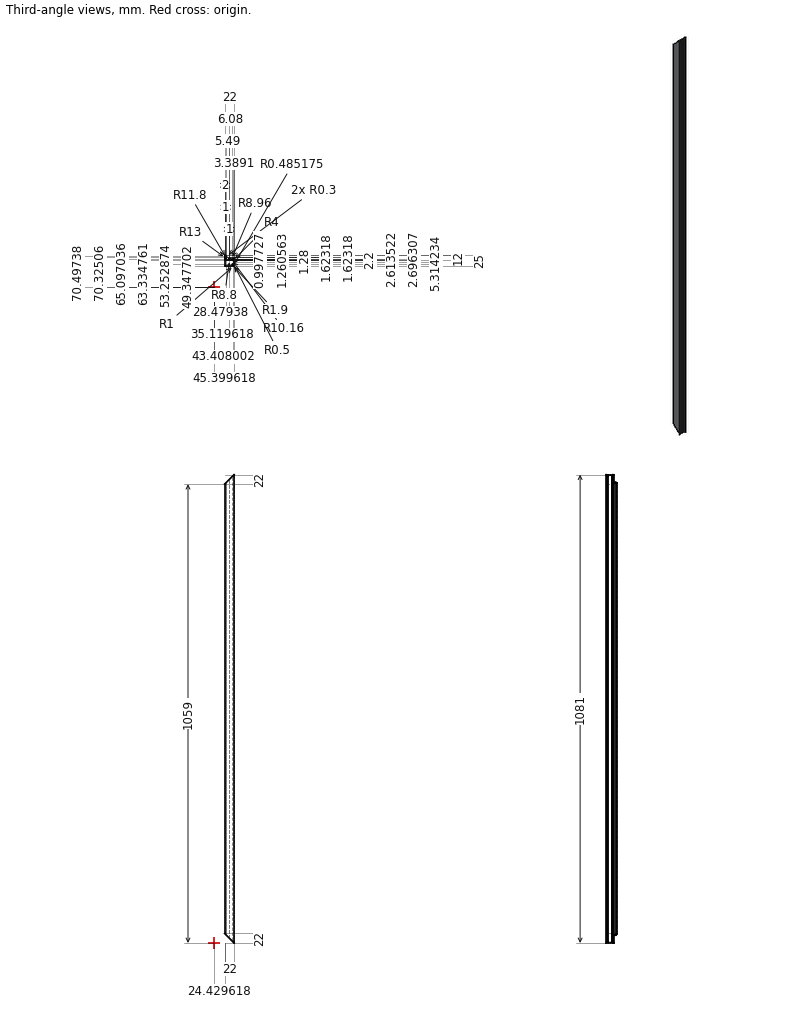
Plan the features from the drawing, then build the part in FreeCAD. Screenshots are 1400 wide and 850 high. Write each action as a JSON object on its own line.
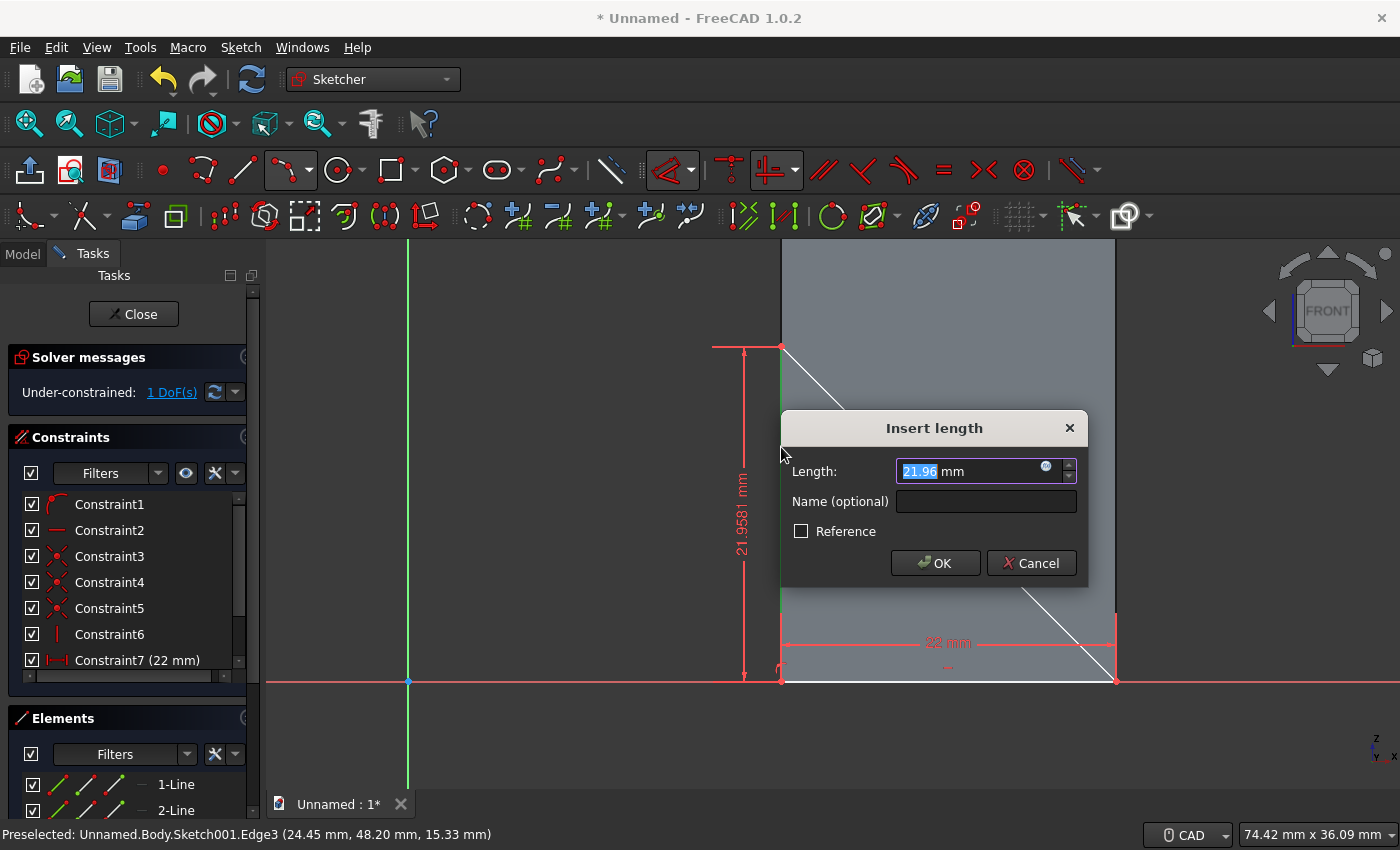
{"action": "type", "text": "22"}
{"action": "key", "text": "Return"}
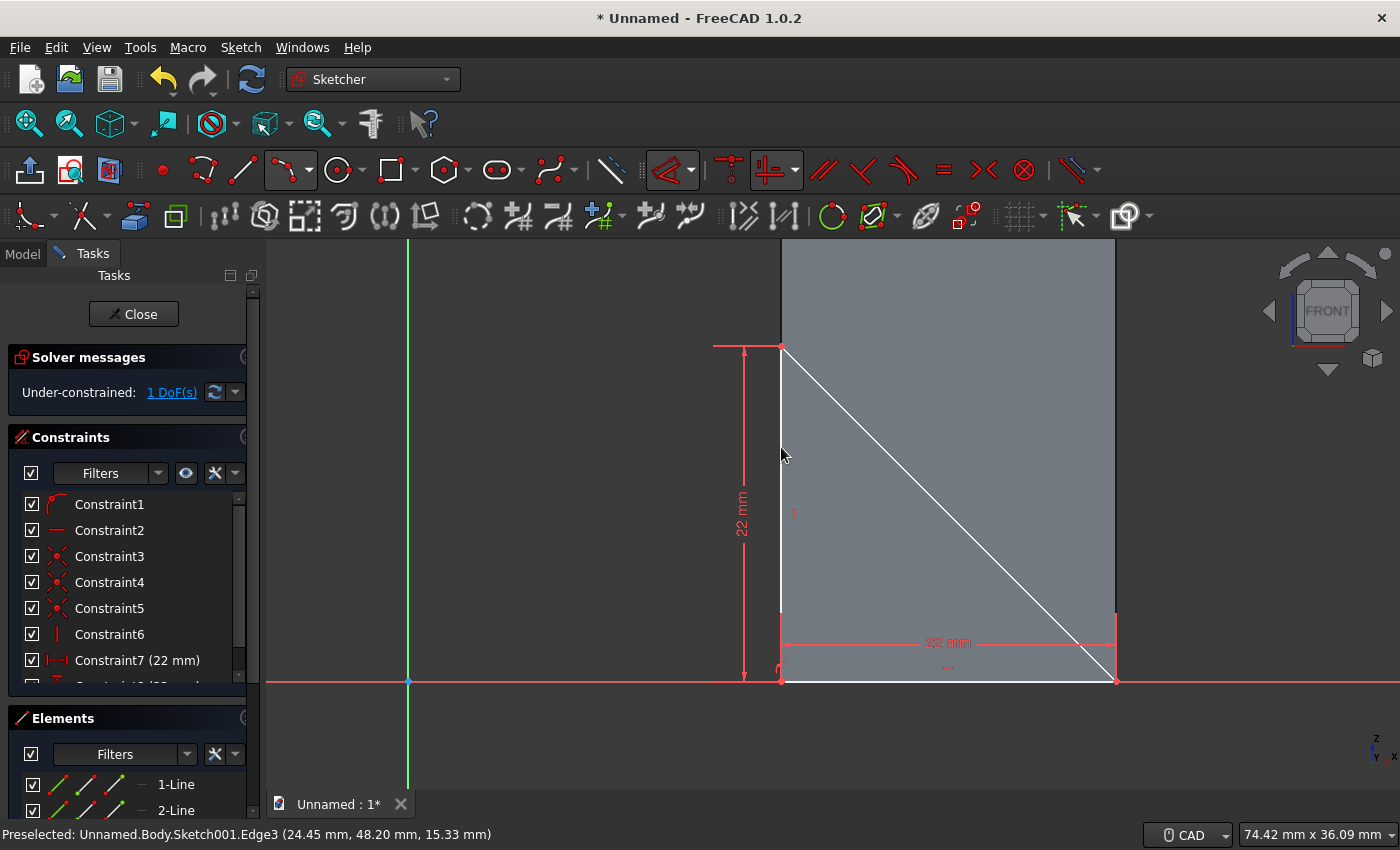
{"action": "left_click", "coordinate": [781, 682]}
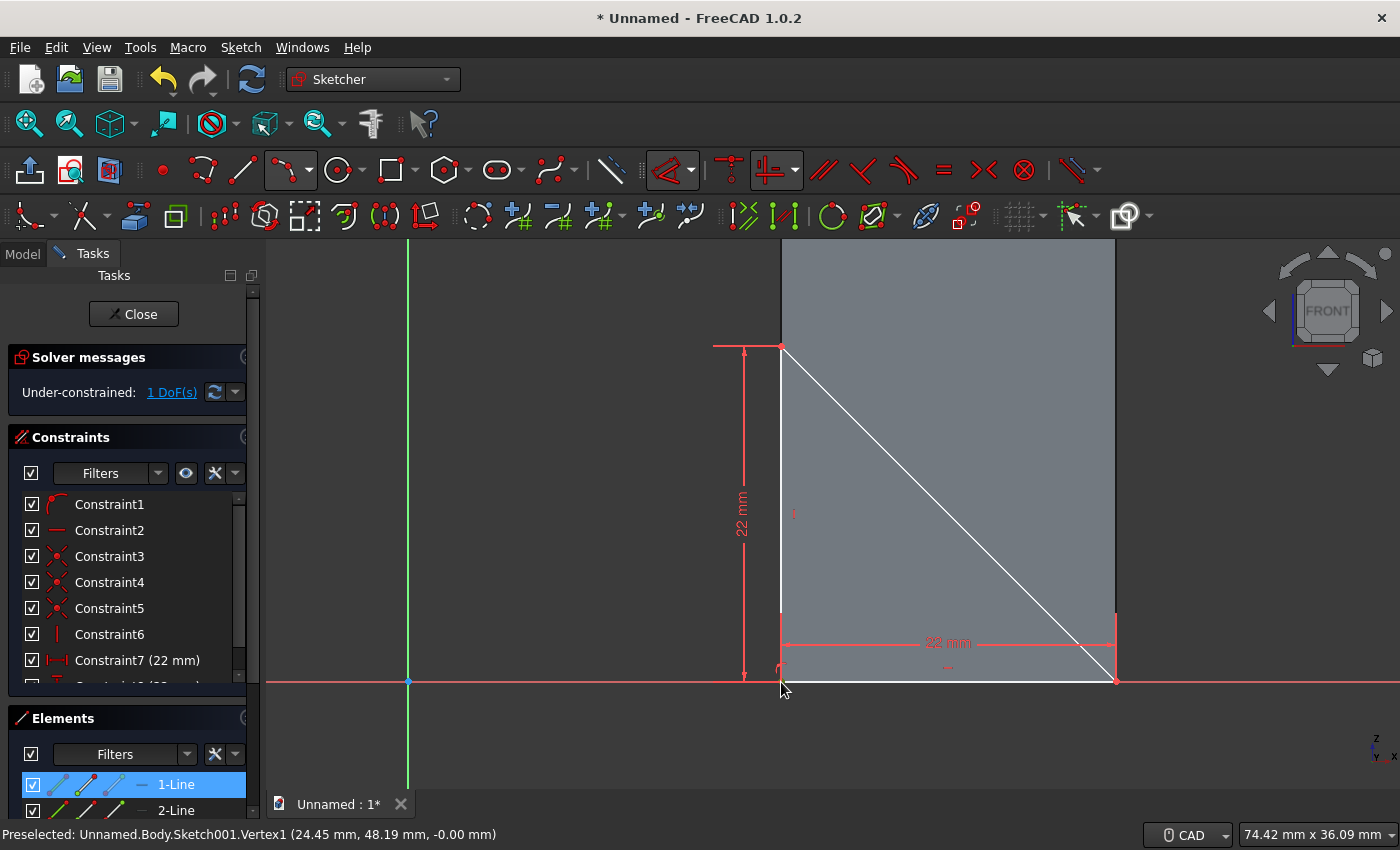
{"action": "left_click", "coordinate": [694, 170]}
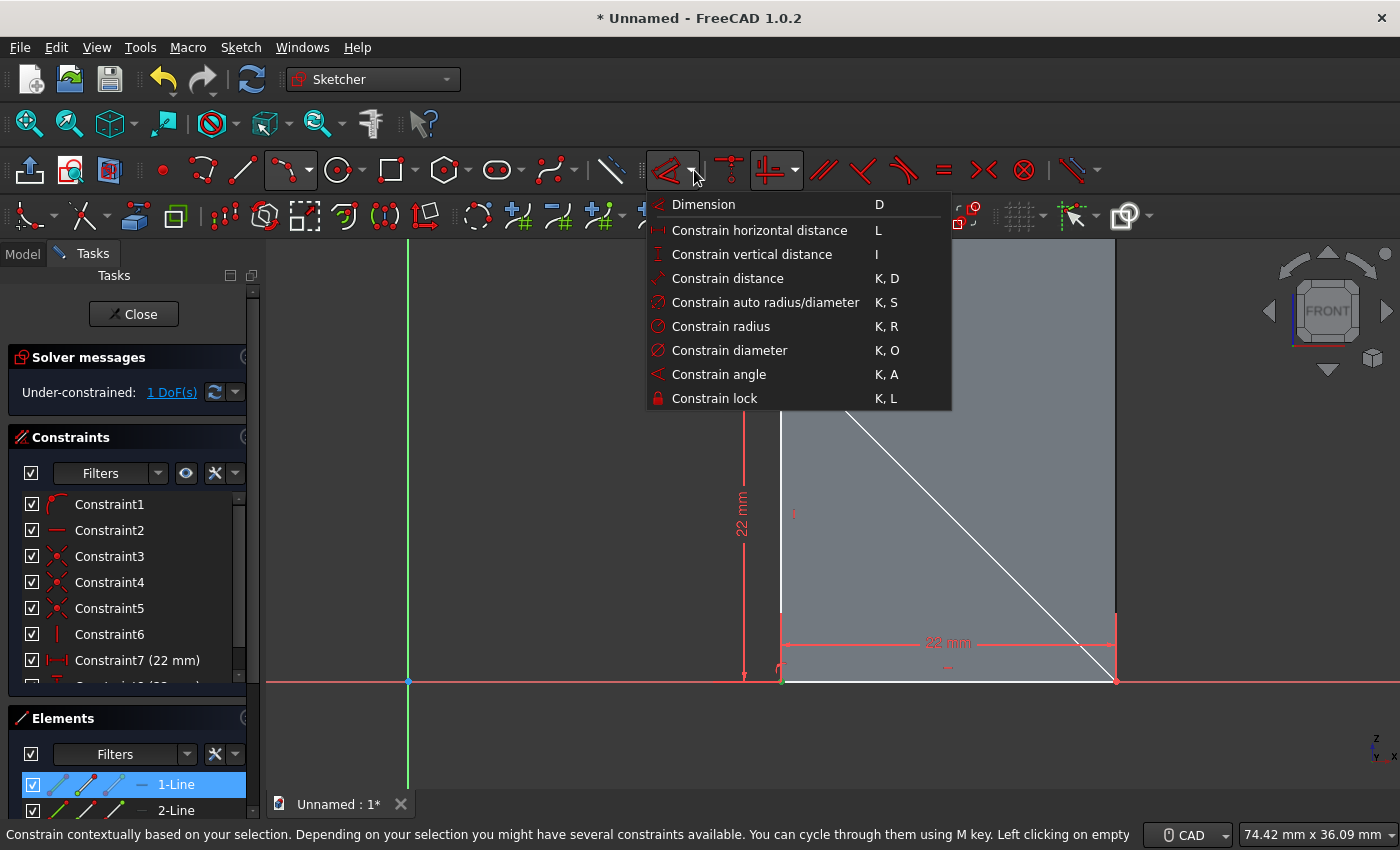
{"action": "left_click", "coordinate": [799, 230]}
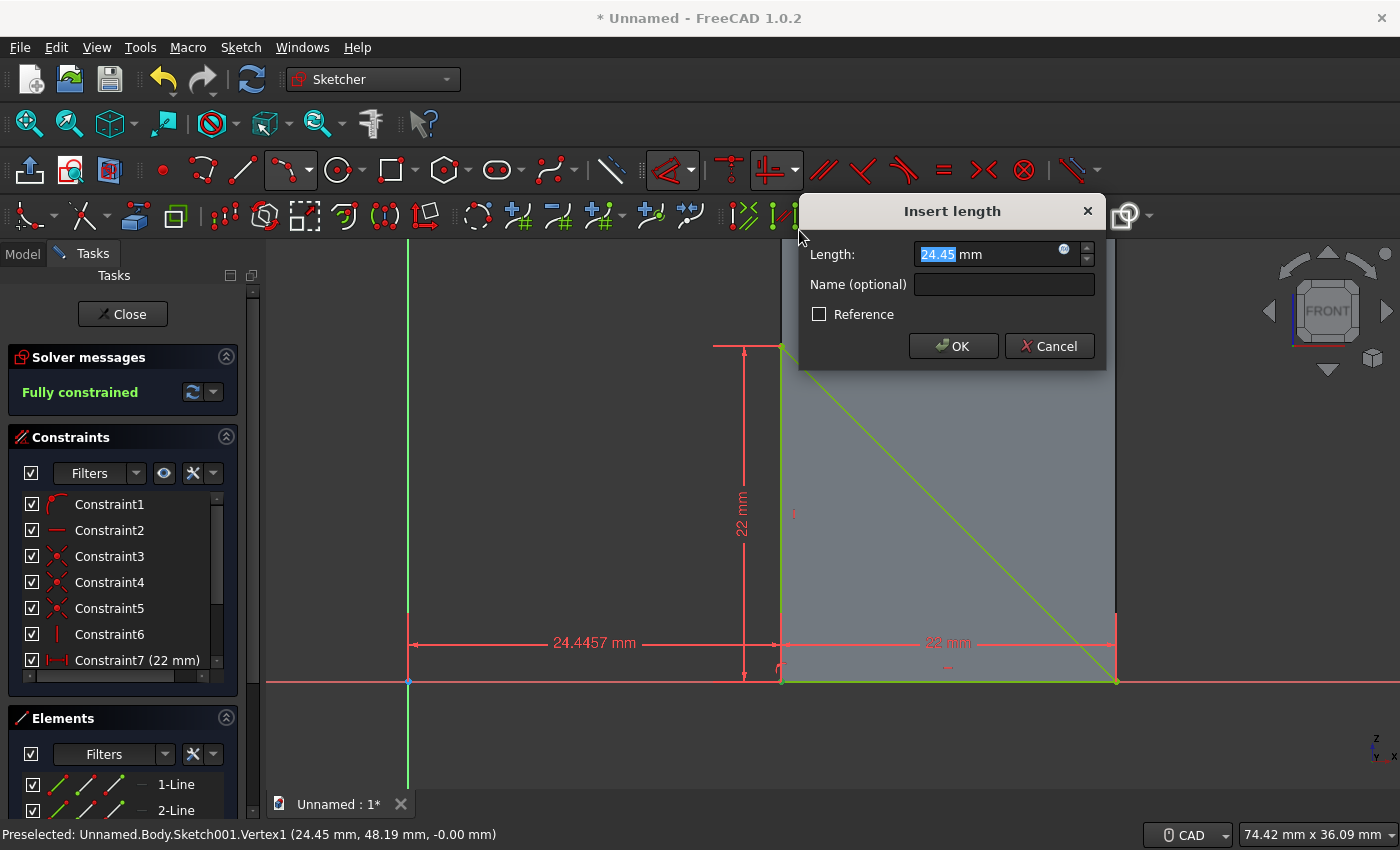
{"action": "type", "text": "24.429618"}
{"action": "key", "text": "Return"}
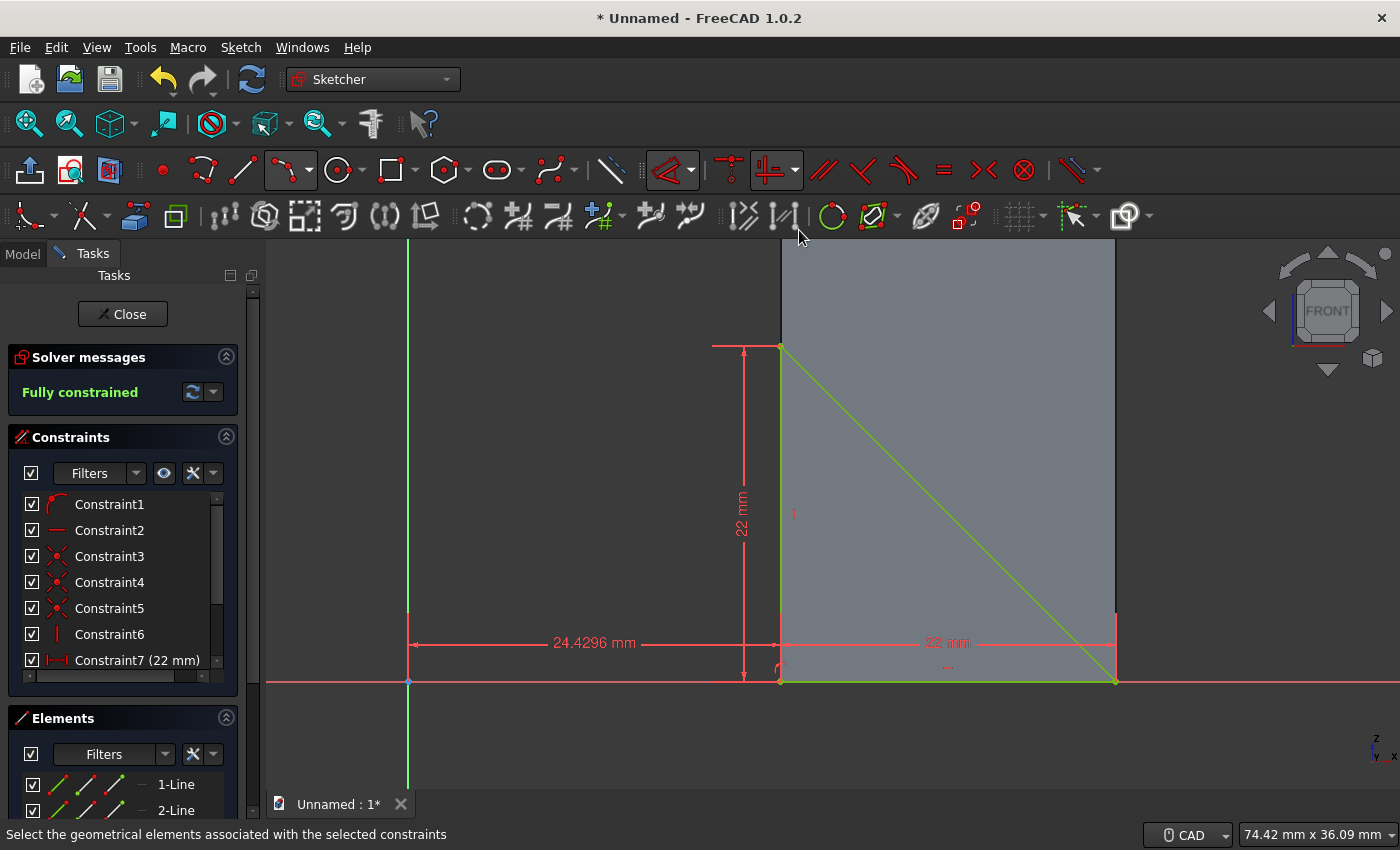
{"action": "left_click", "coordinate": [123, 314]}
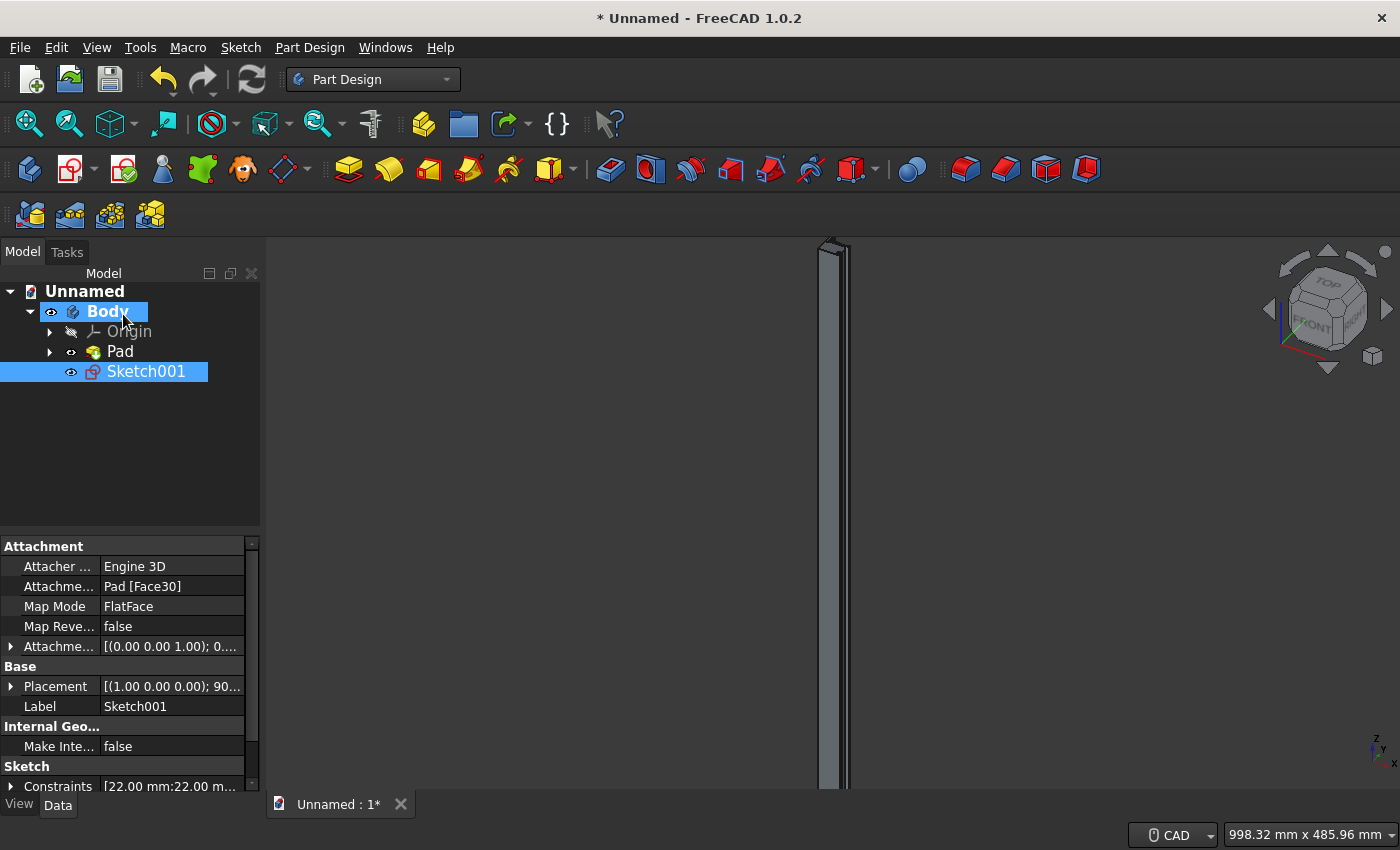
{"action": "left_click", "coordinate": [612, 170]}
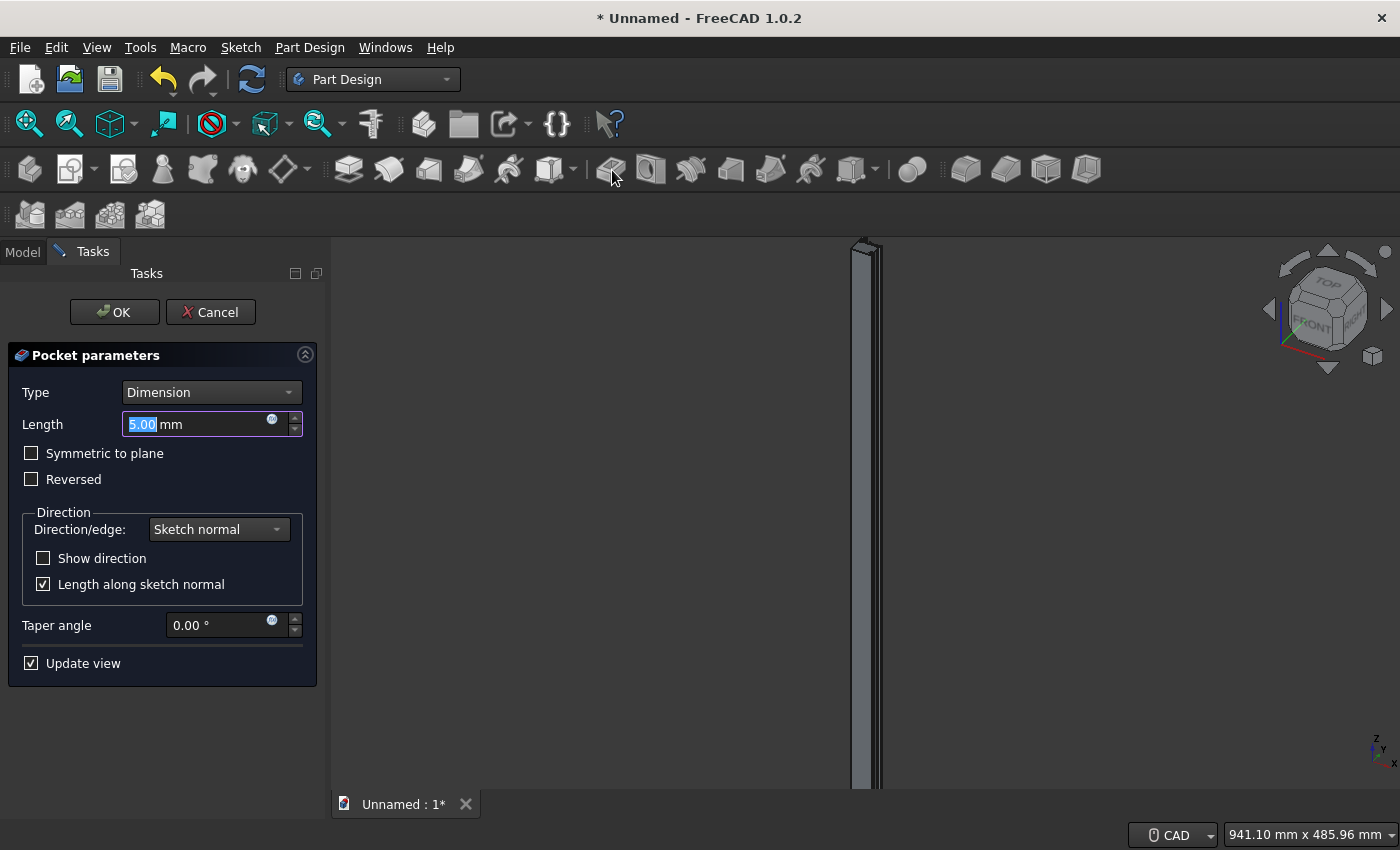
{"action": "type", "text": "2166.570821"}
{"action": "key", "text": "Tab"}